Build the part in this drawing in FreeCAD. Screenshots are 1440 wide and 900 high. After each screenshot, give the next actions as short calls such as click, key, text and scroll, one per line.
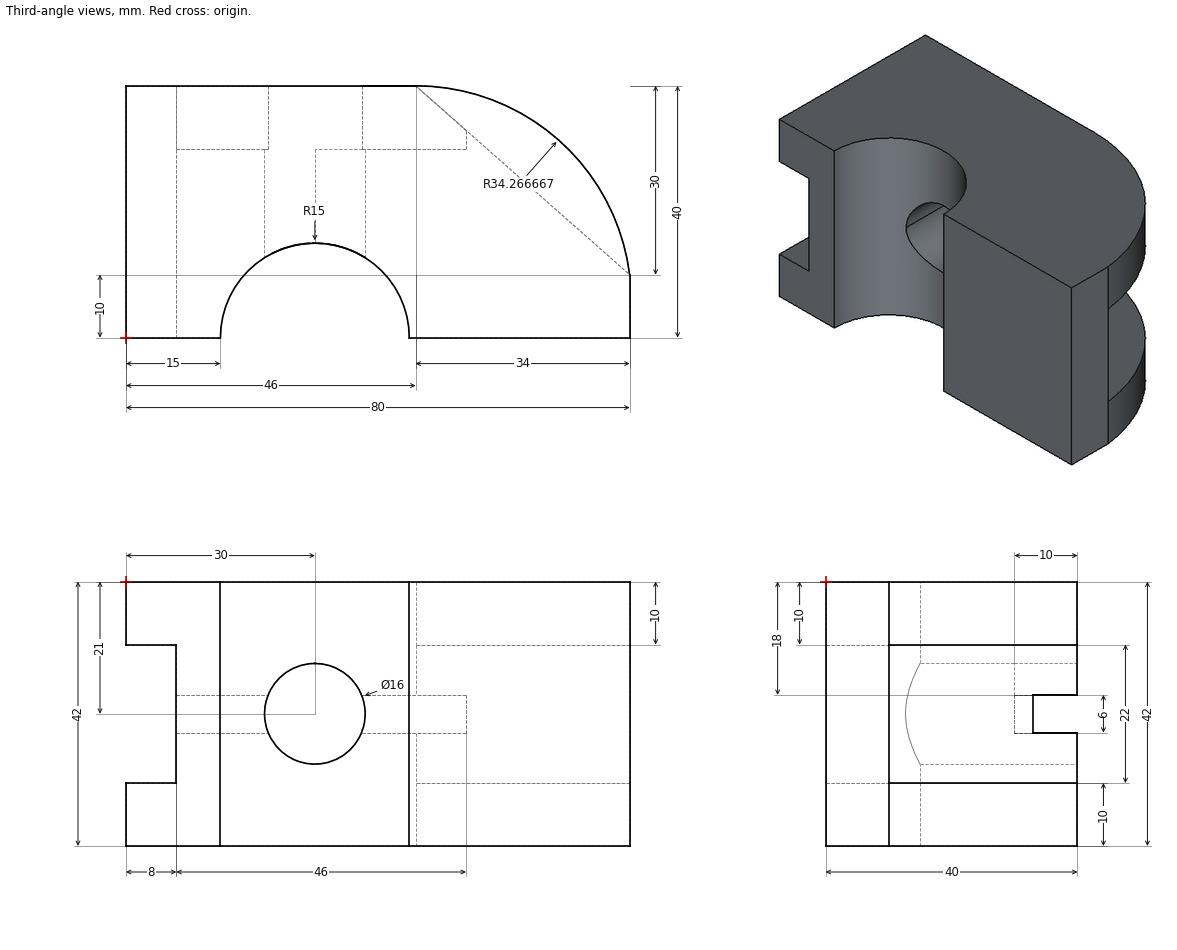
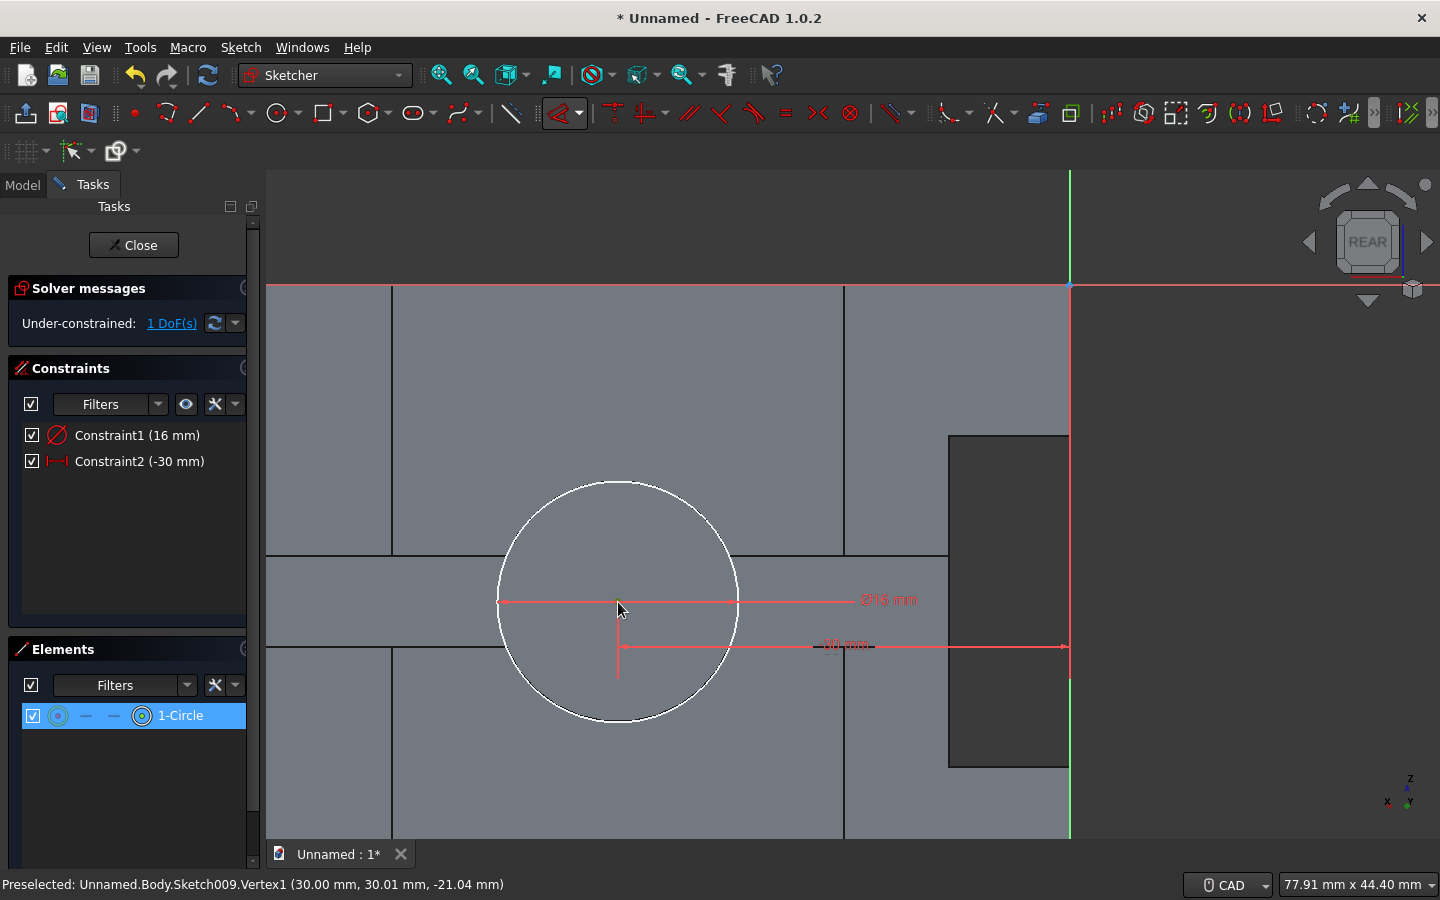
click(582, 114)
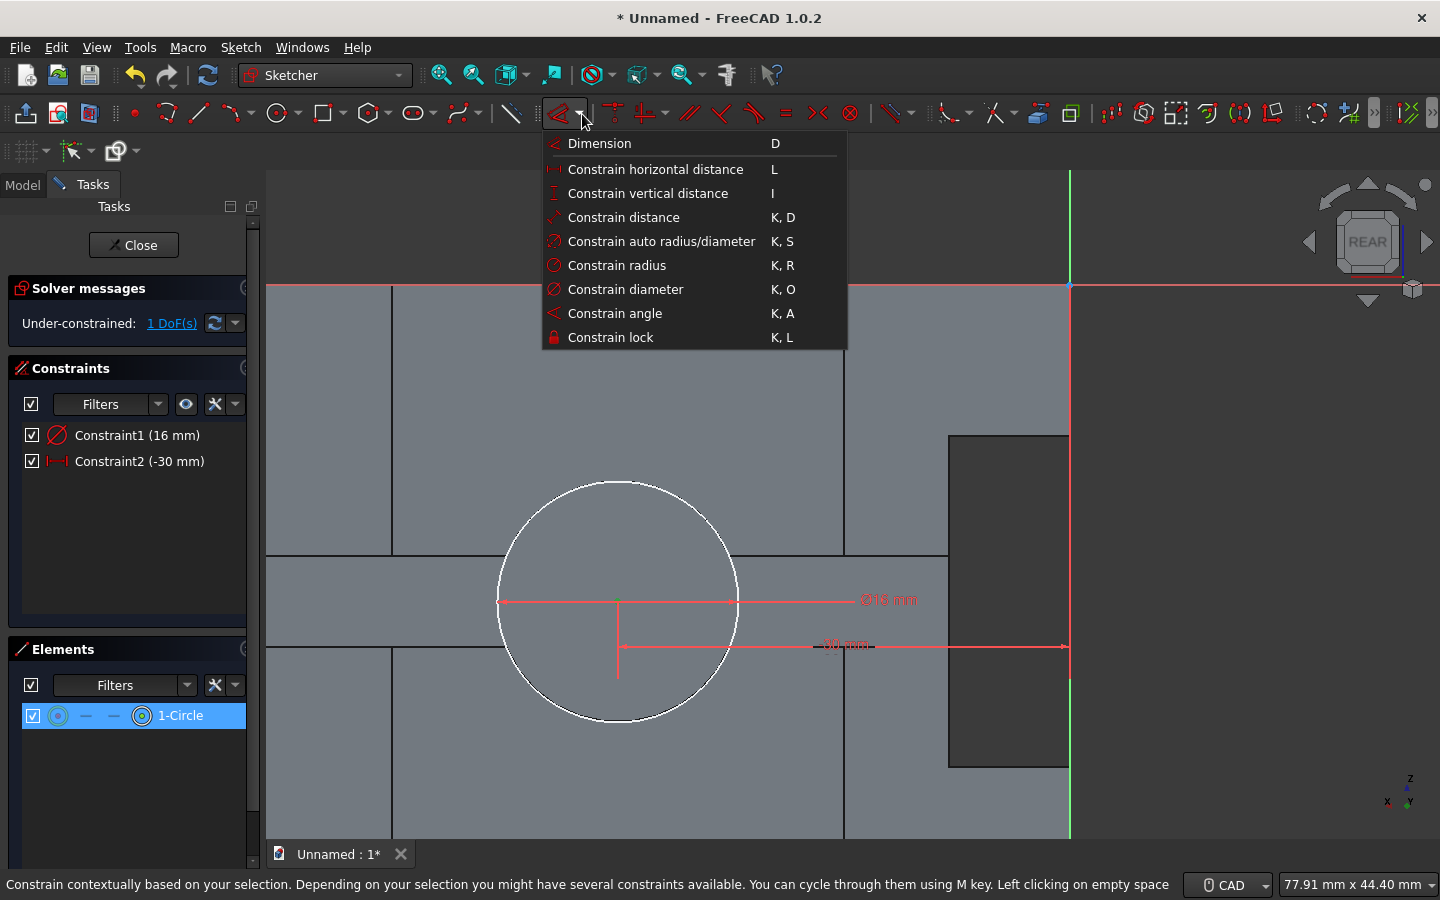
click(695, 193)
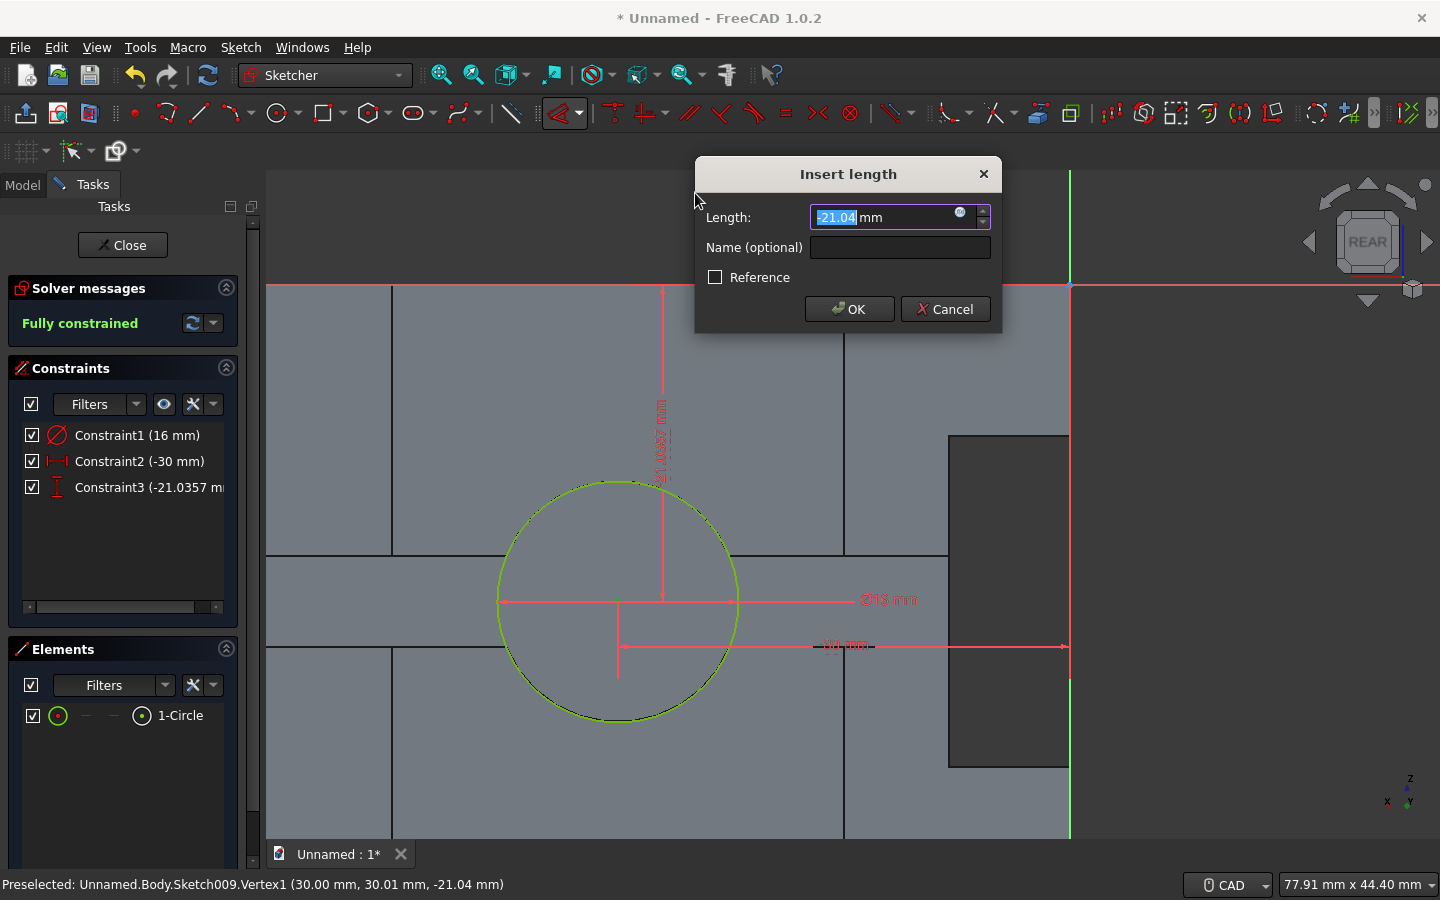
text(-21)
key(Return)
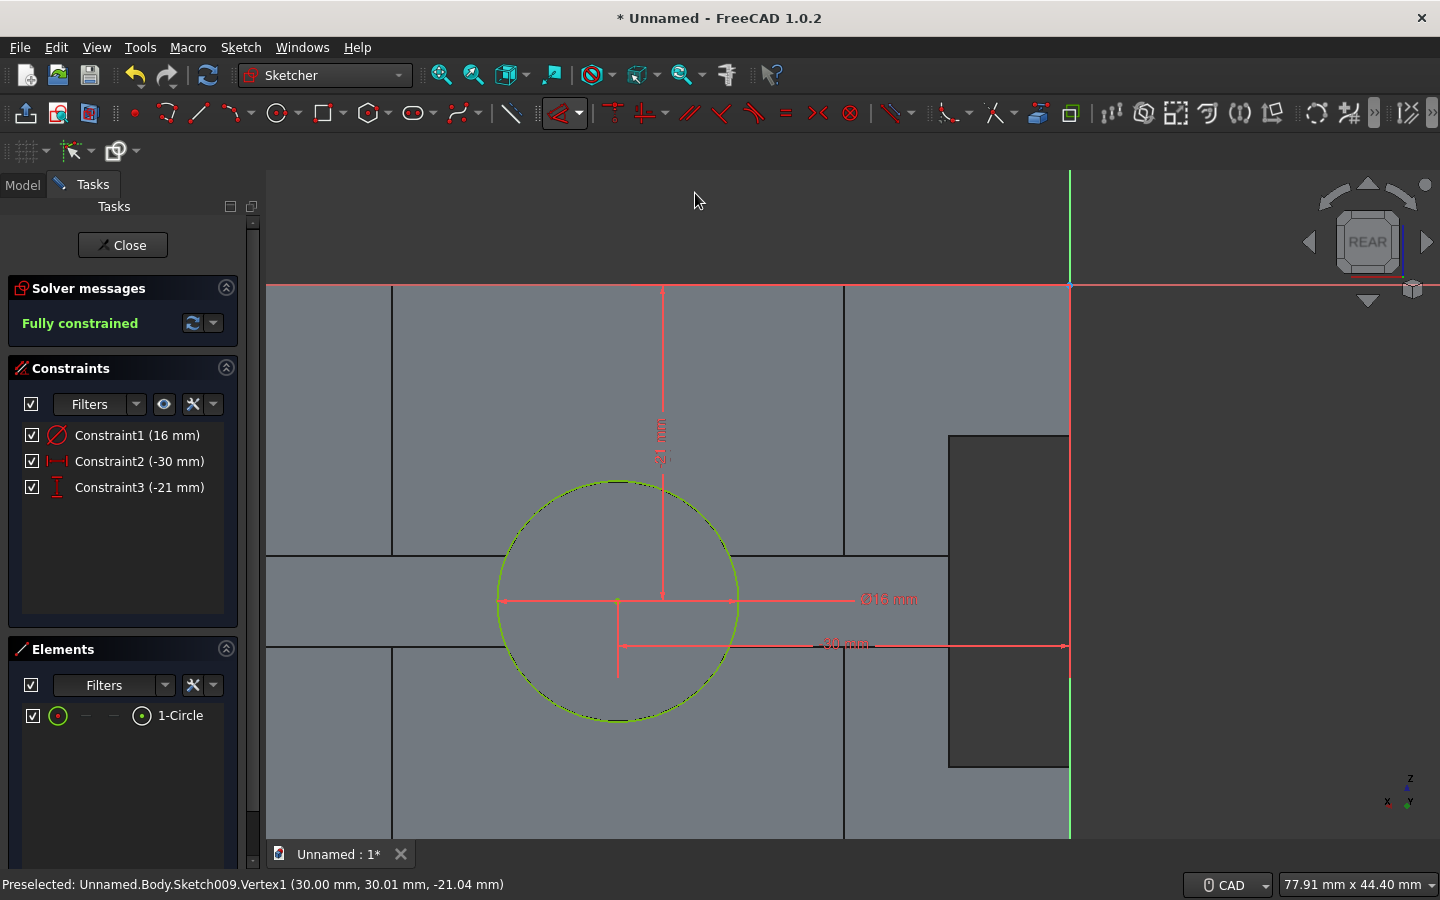
click(123, 245)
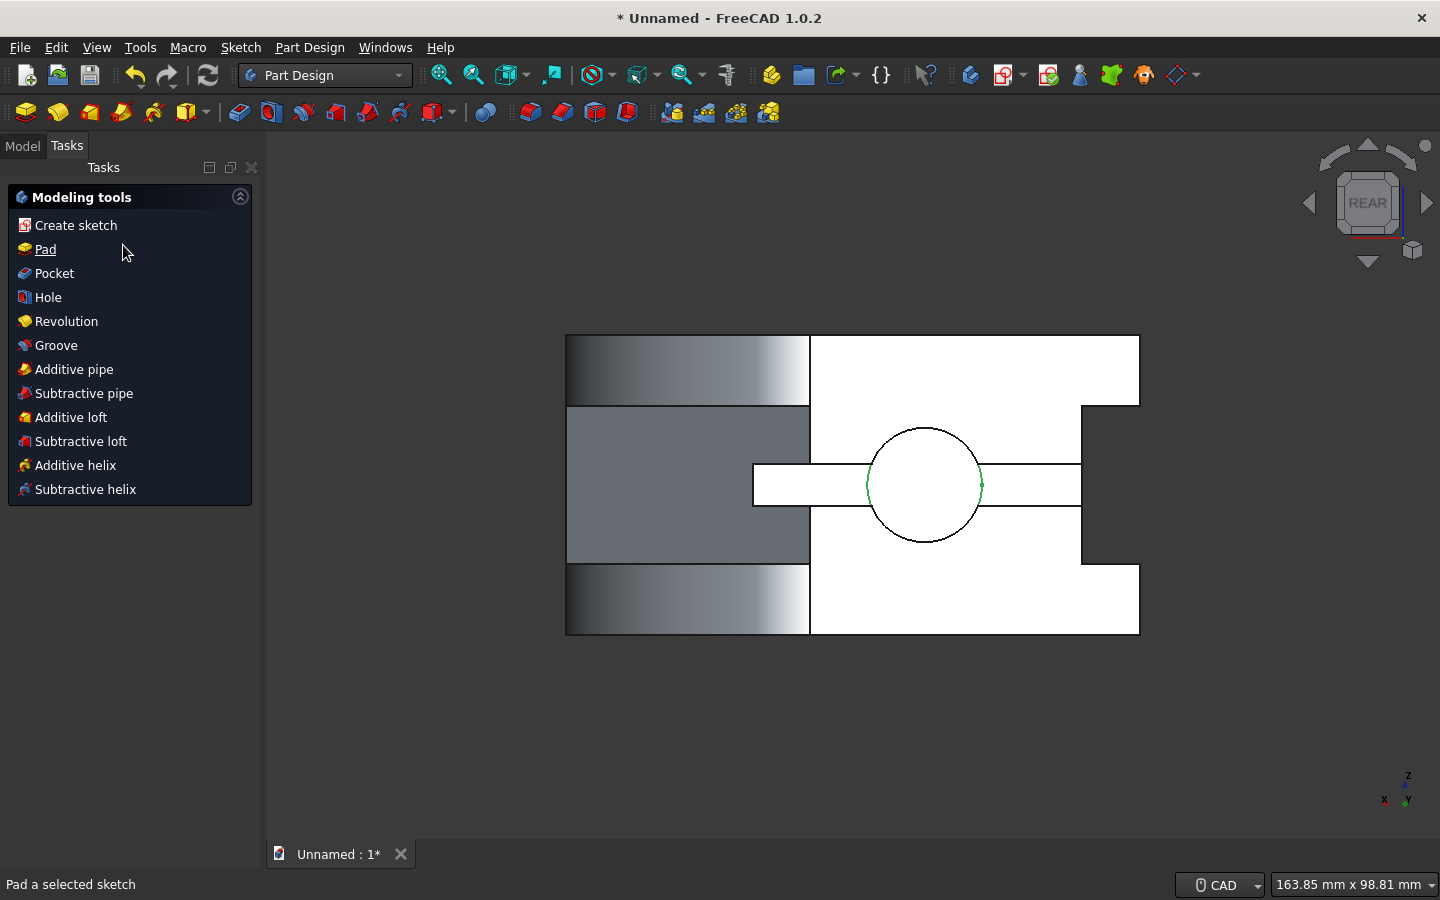
click(240, 112)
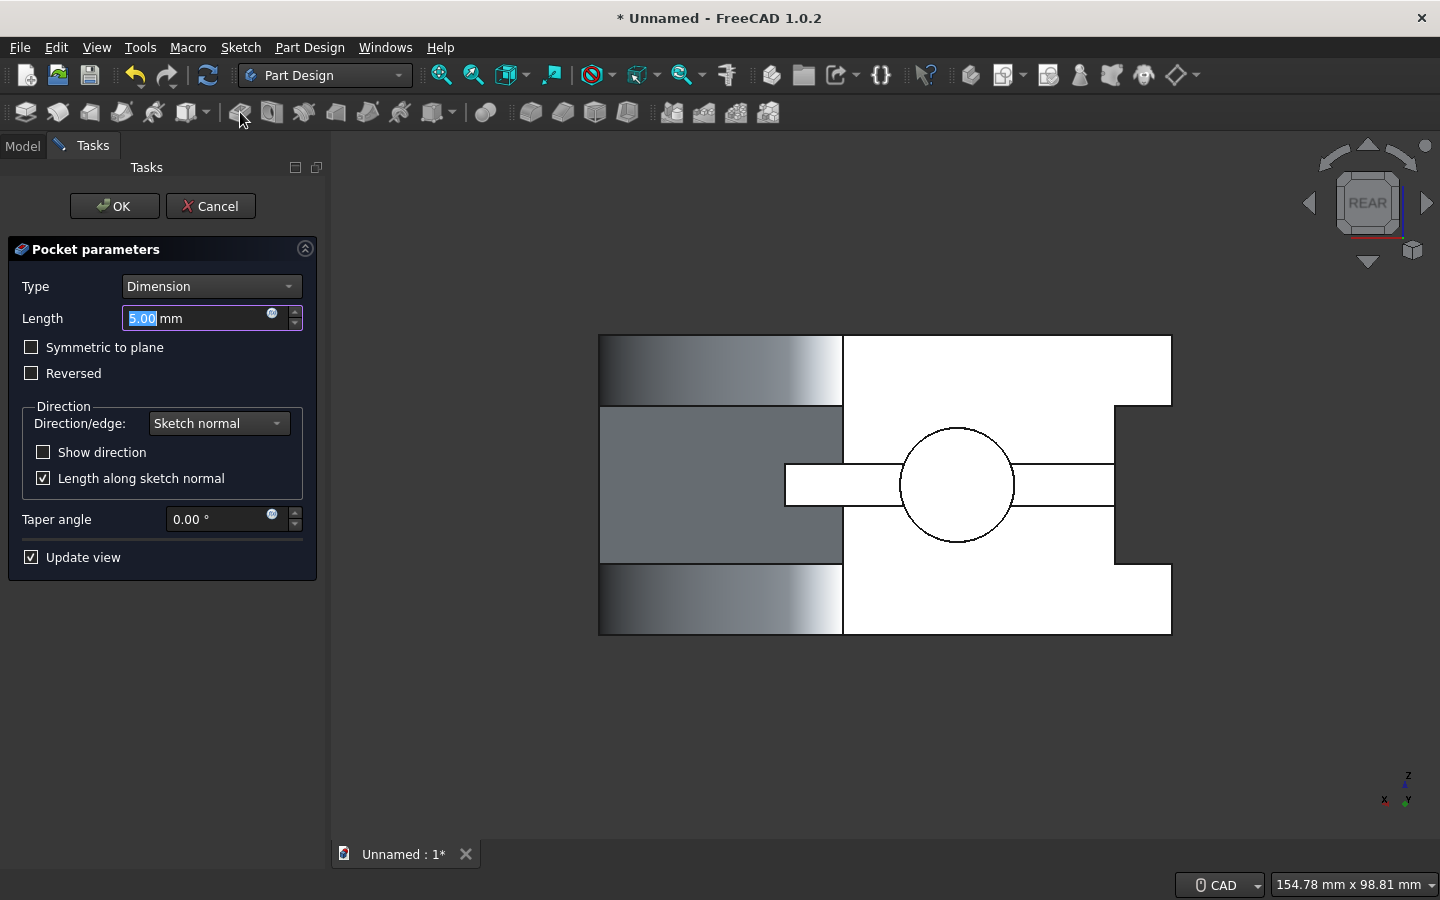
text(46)
key(Tab)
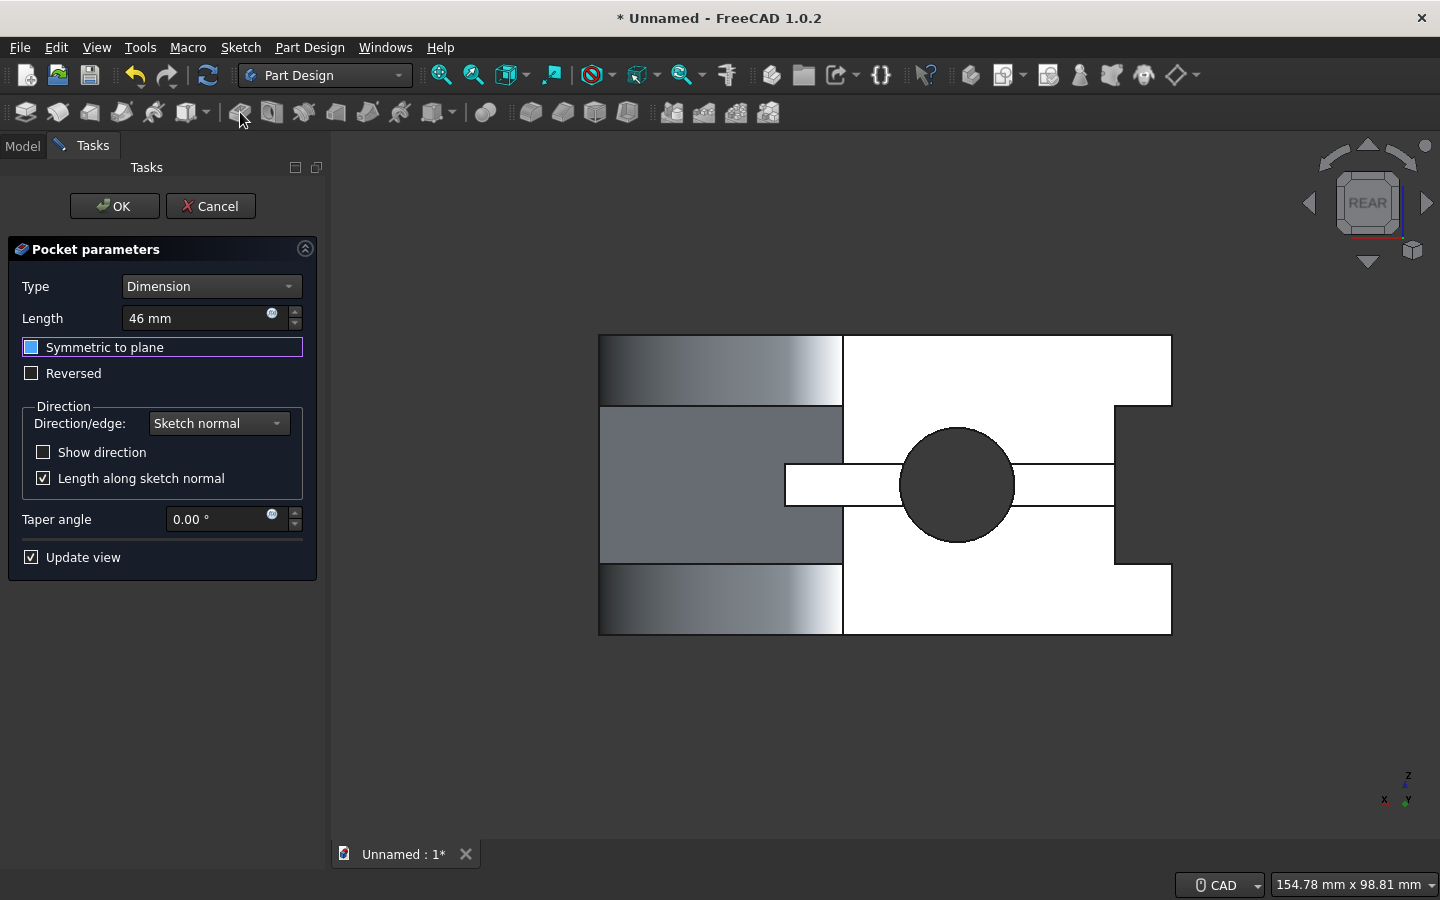
click(115, 206)